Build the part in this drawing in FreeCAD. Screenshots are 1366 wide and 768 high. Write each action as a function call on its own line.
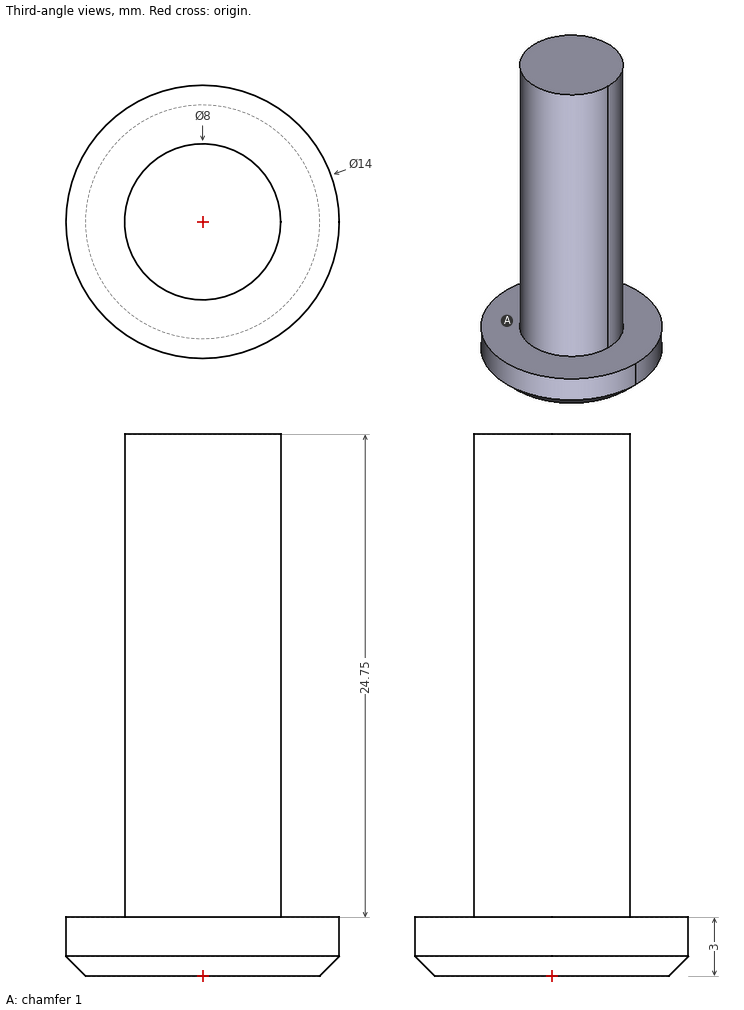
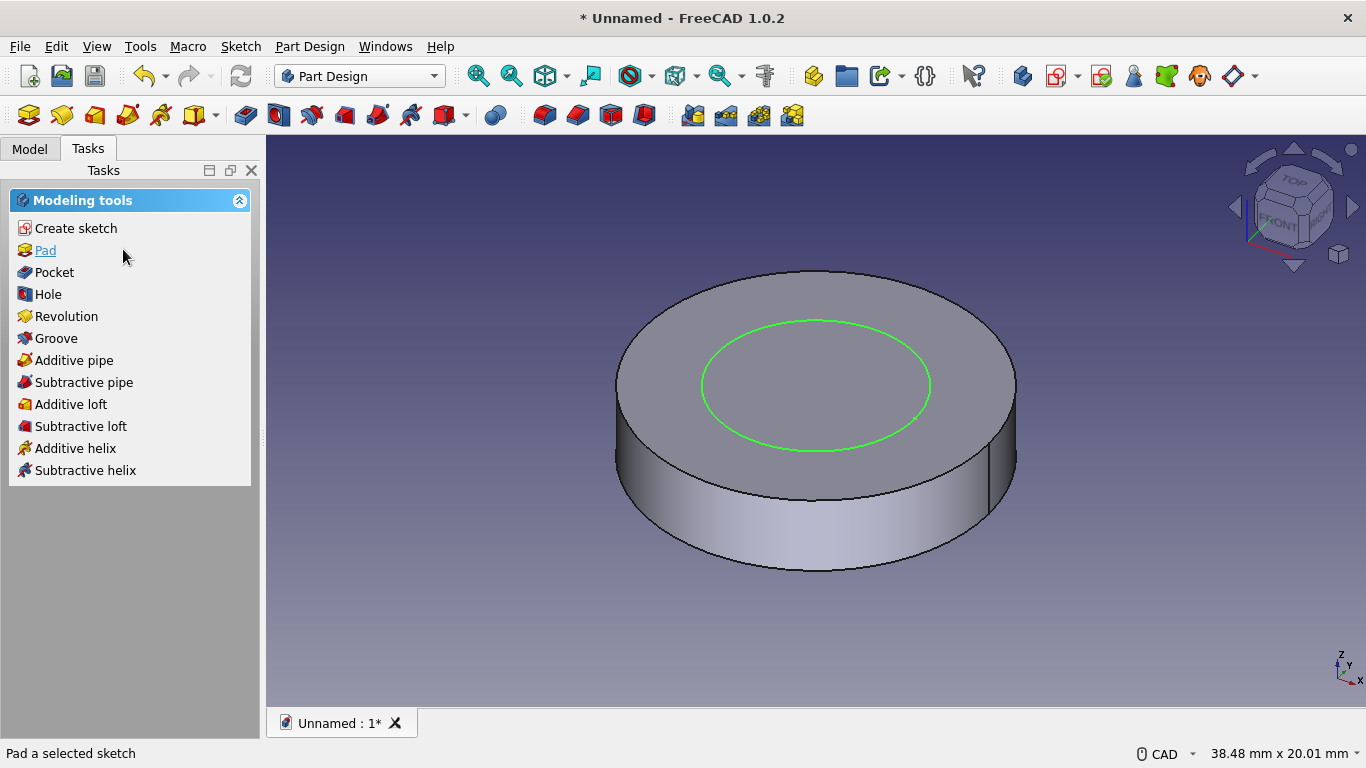
click(29, 116)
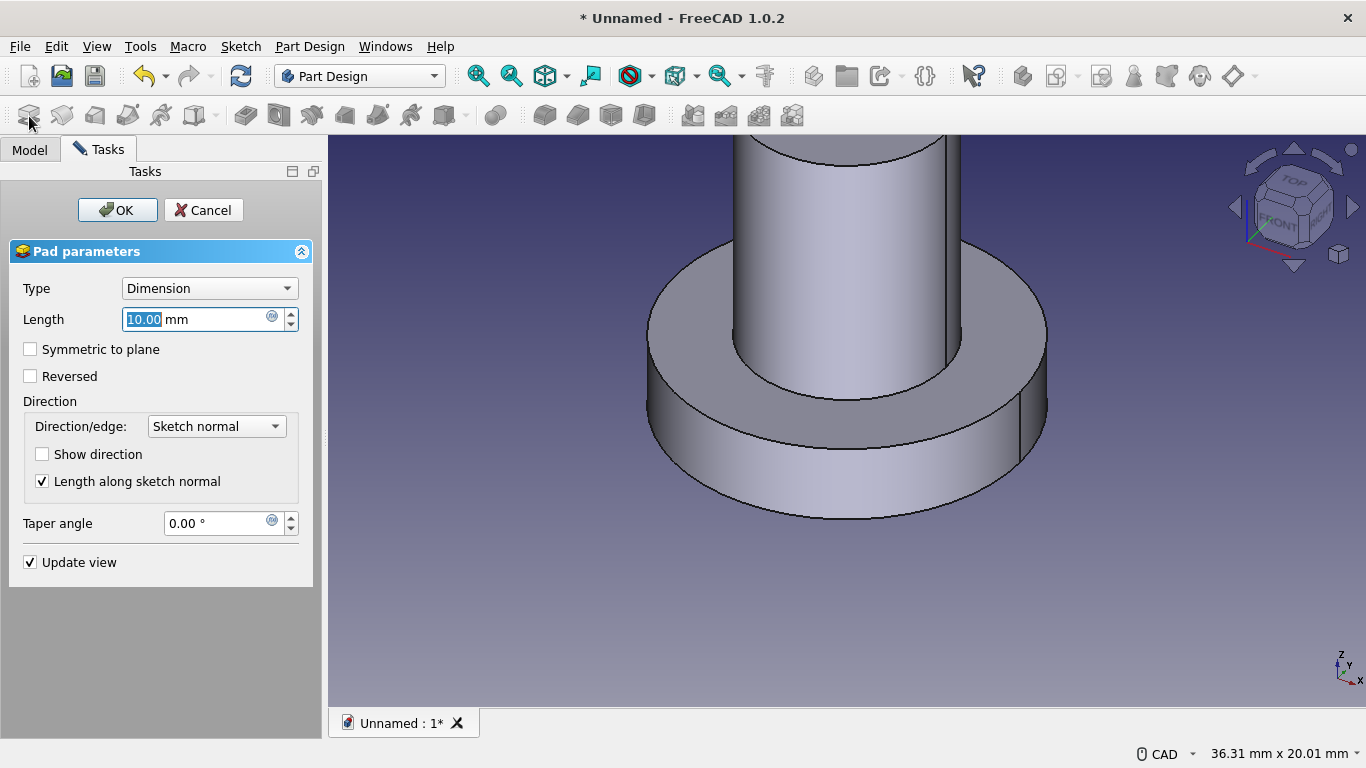
text(24.75)
key(Tab)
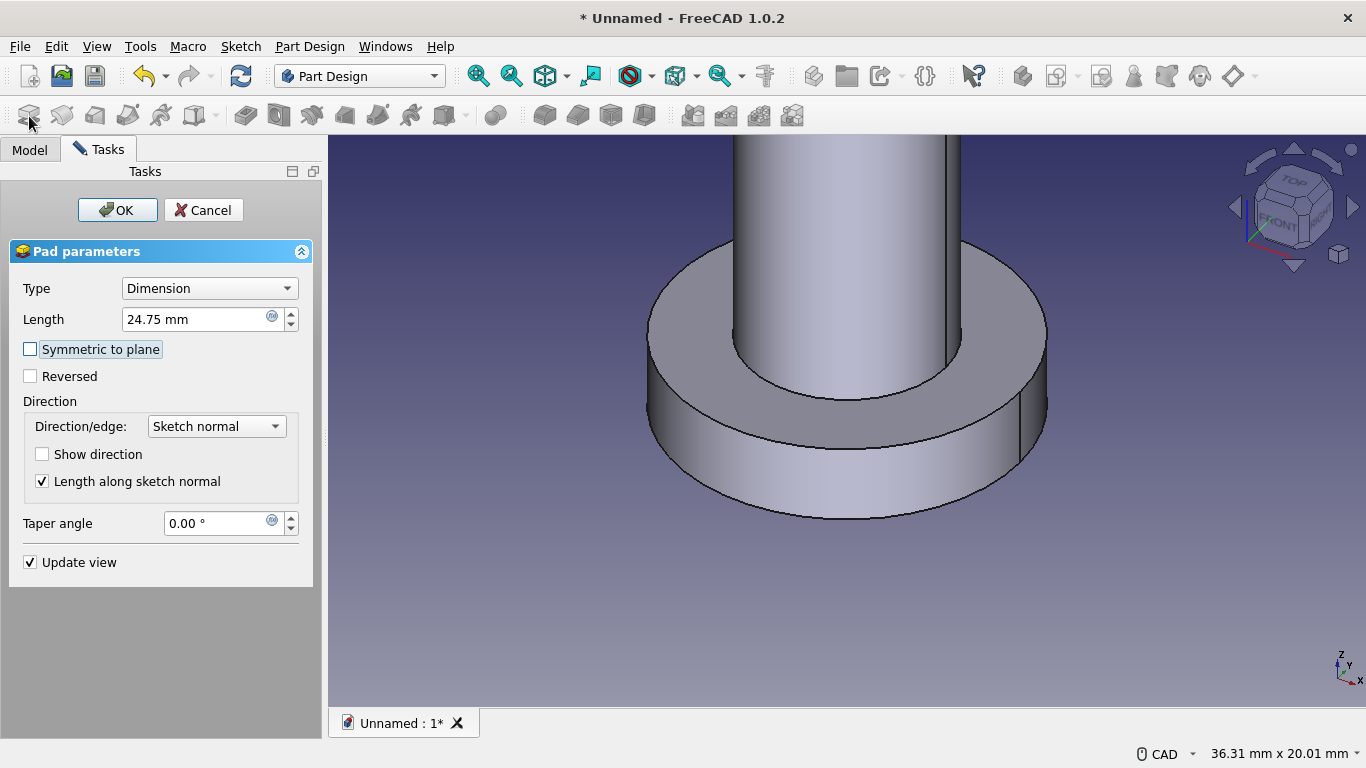
click(118, 210)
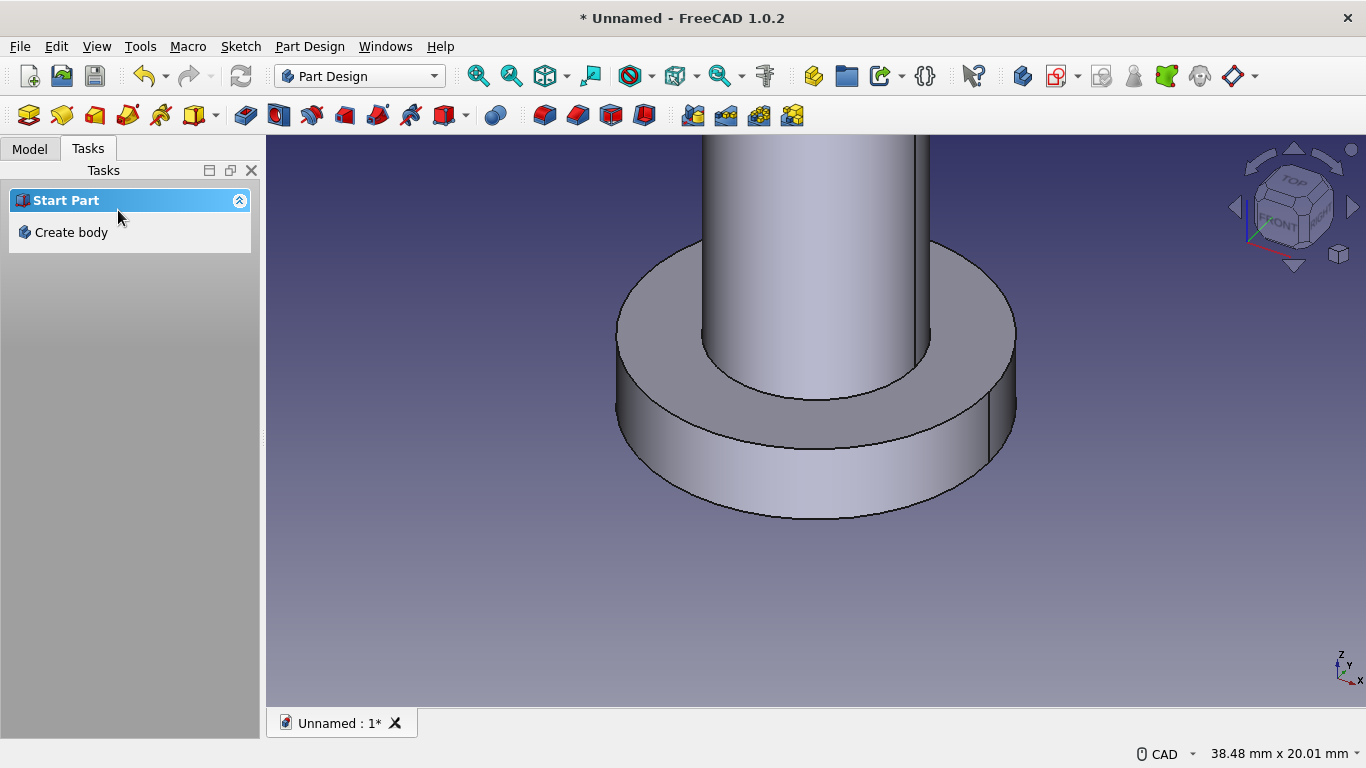
click(479, 76)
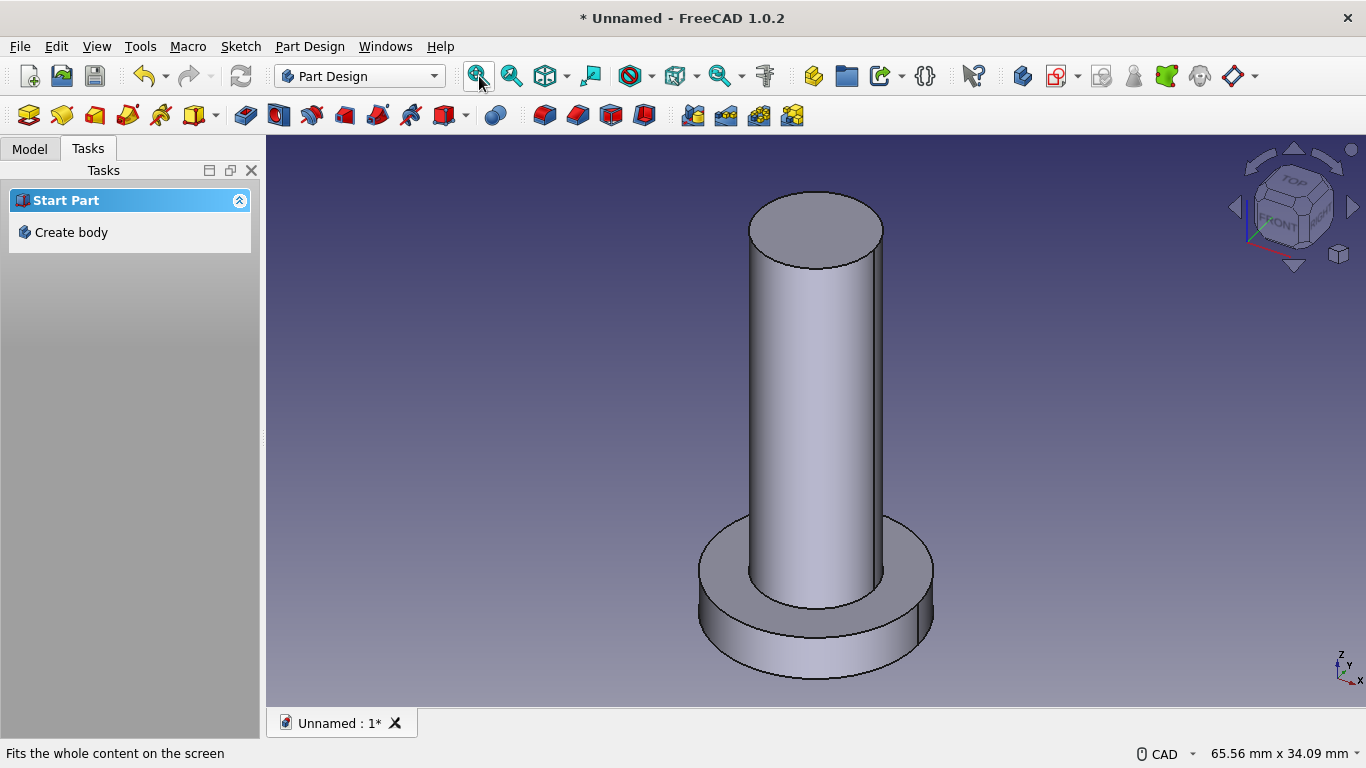
key(0)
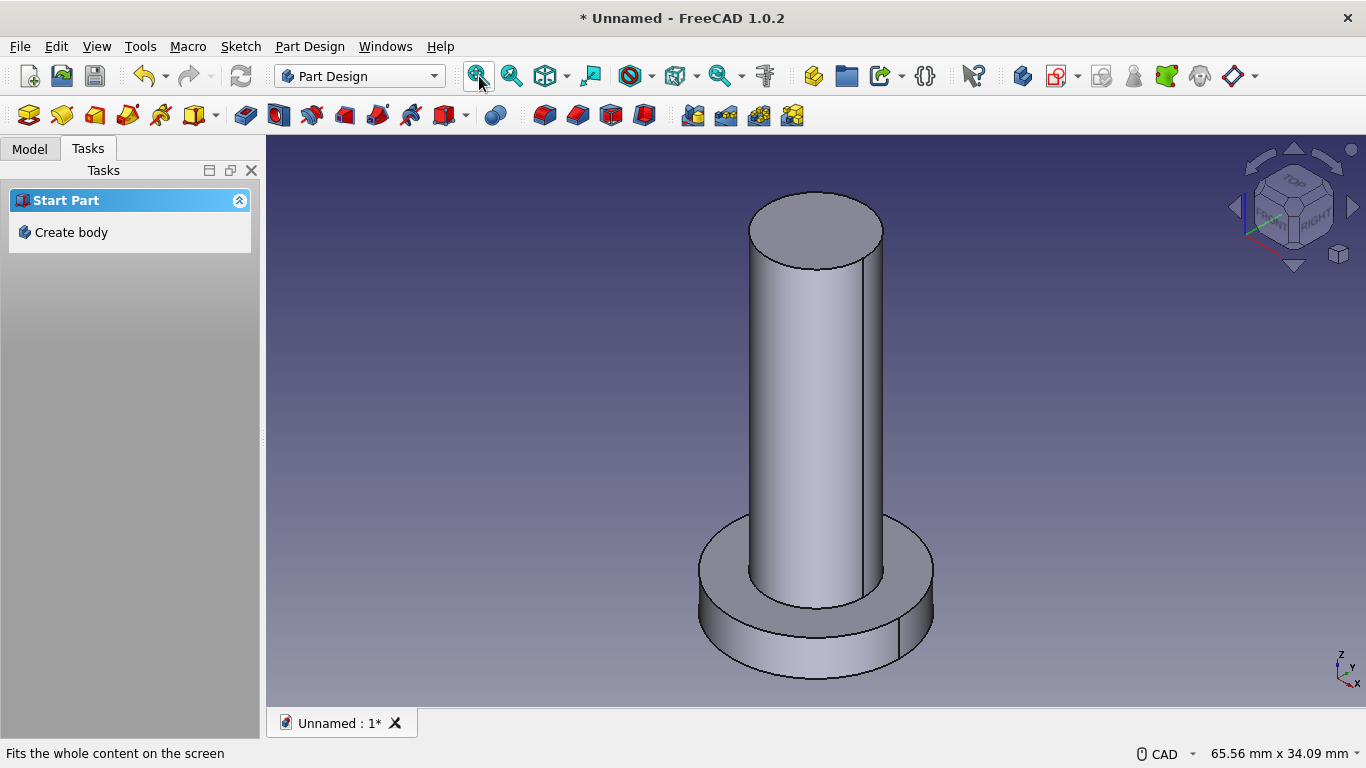
click(479, 76)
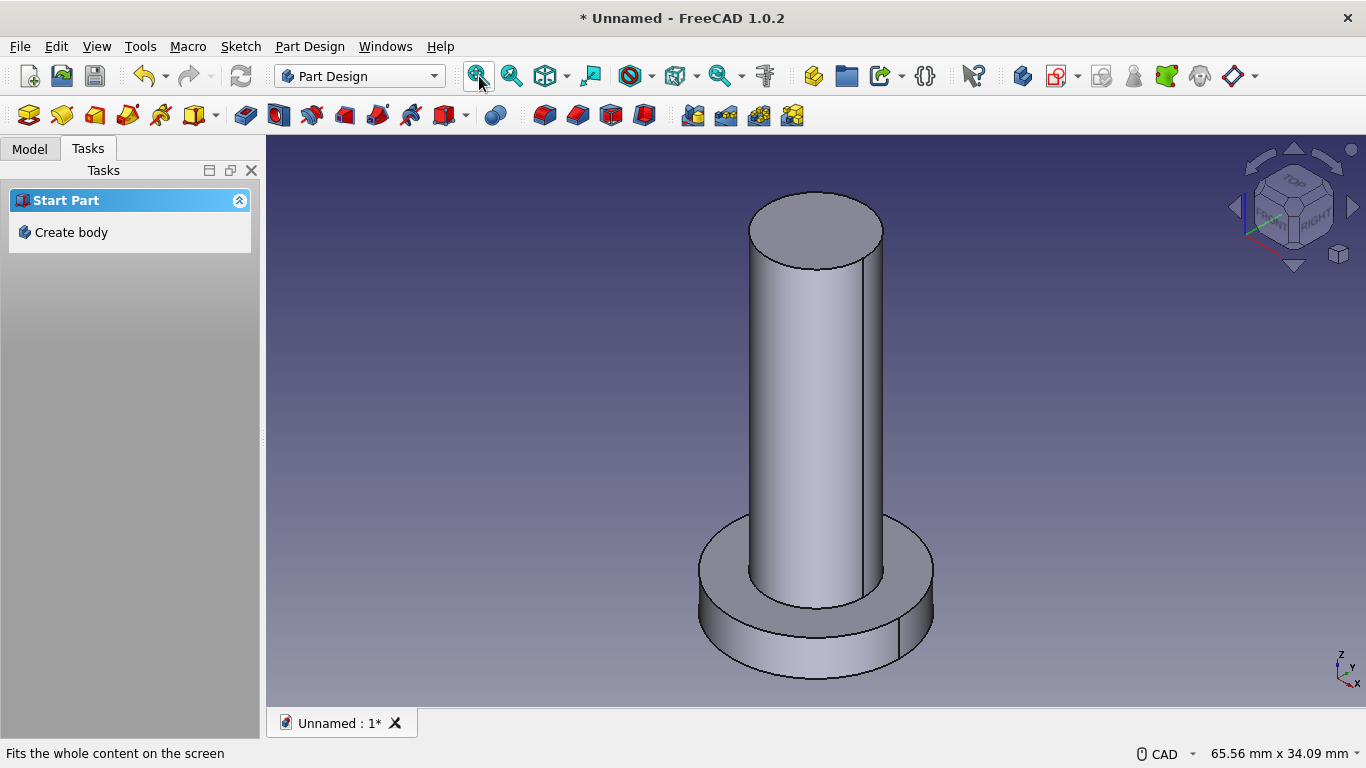
click(711, 641)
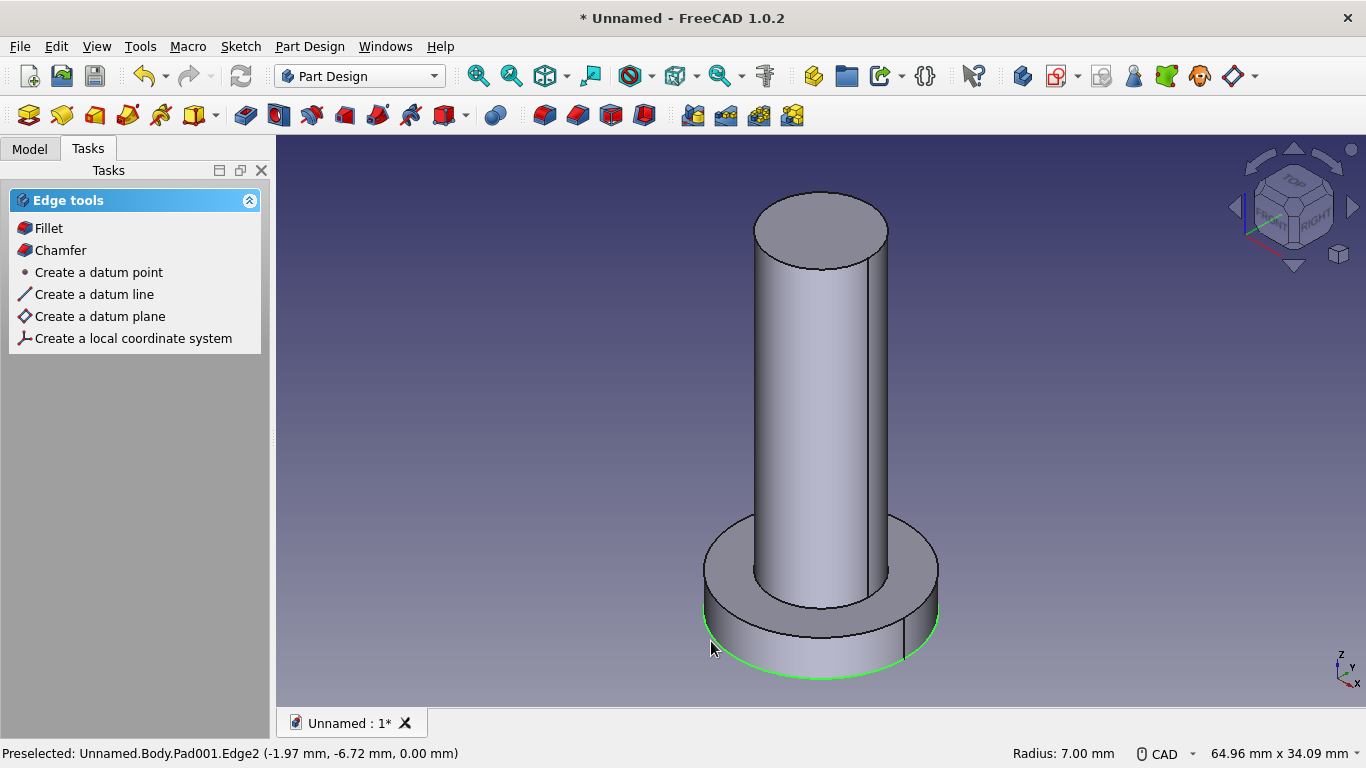
click(578, 116)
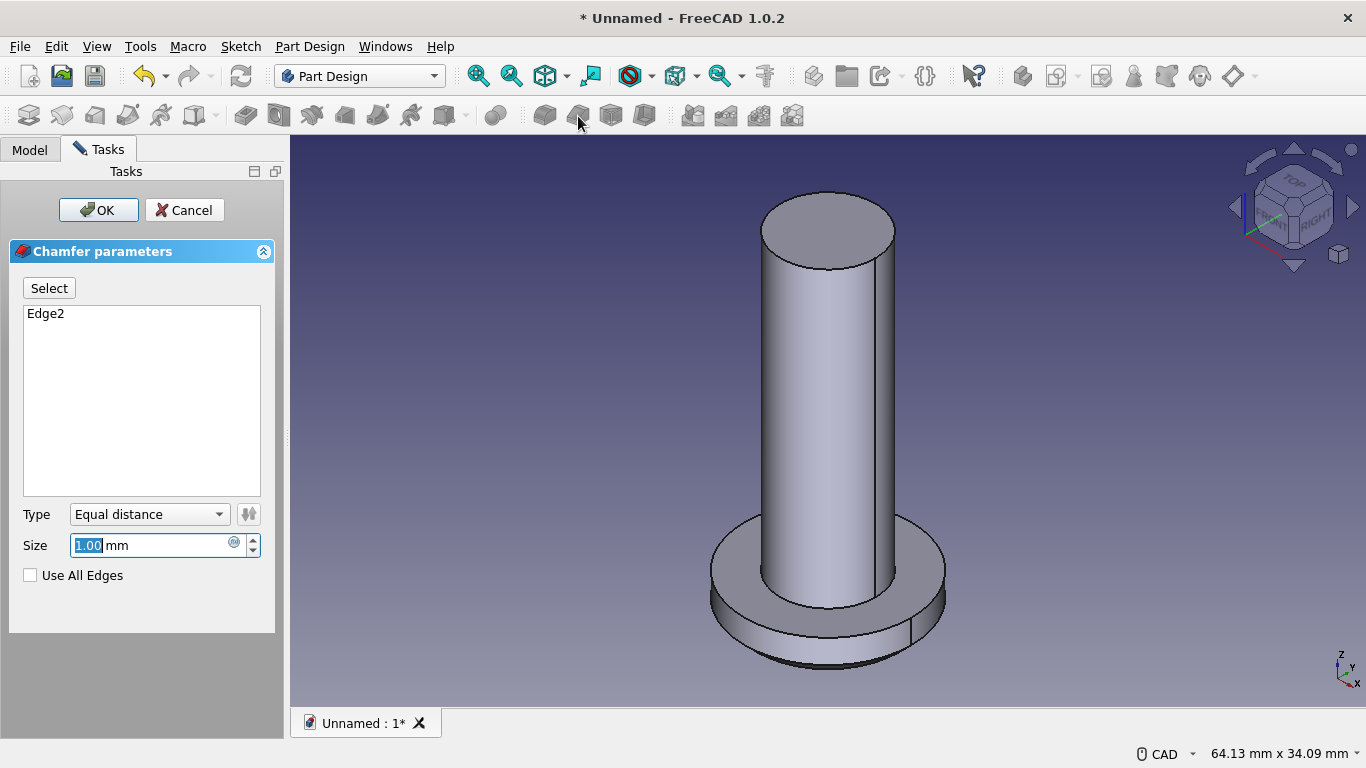
text(1)
key(Tab)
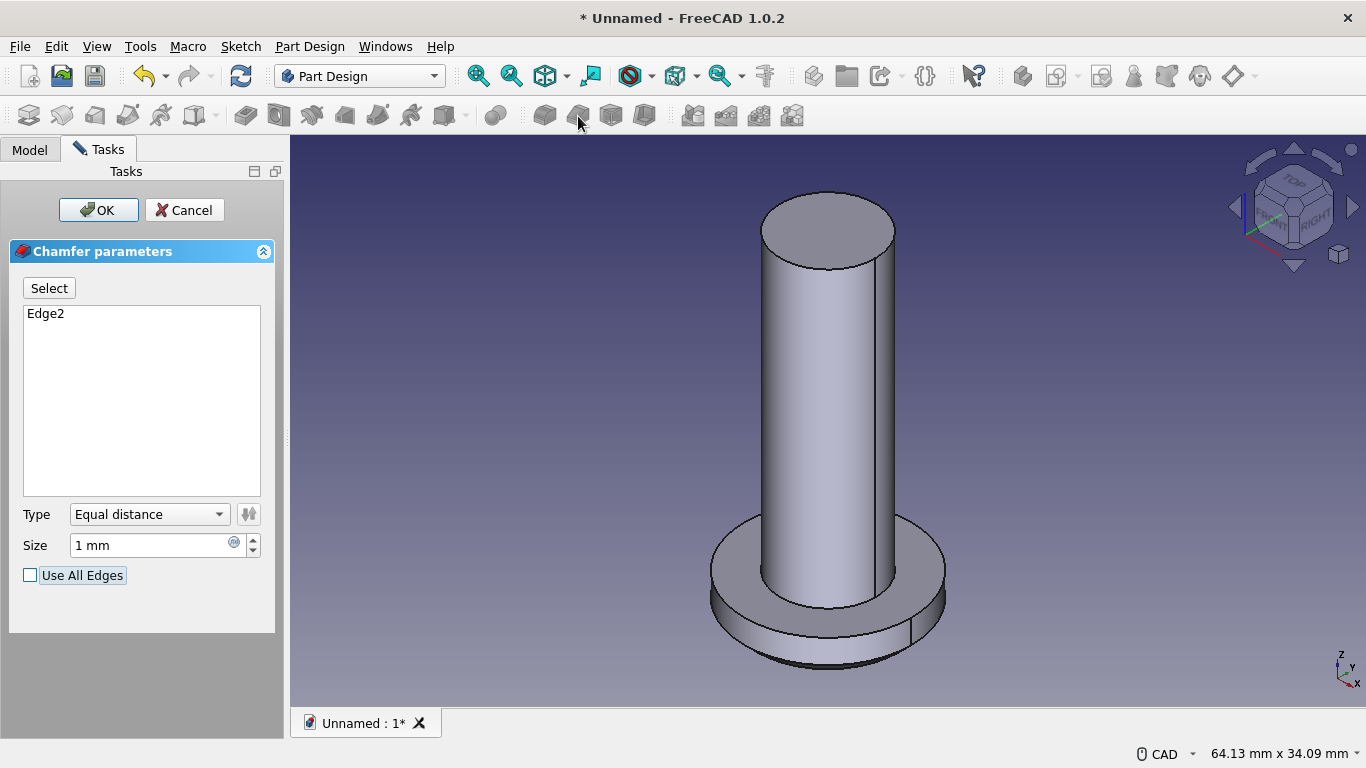
click(99, 210)